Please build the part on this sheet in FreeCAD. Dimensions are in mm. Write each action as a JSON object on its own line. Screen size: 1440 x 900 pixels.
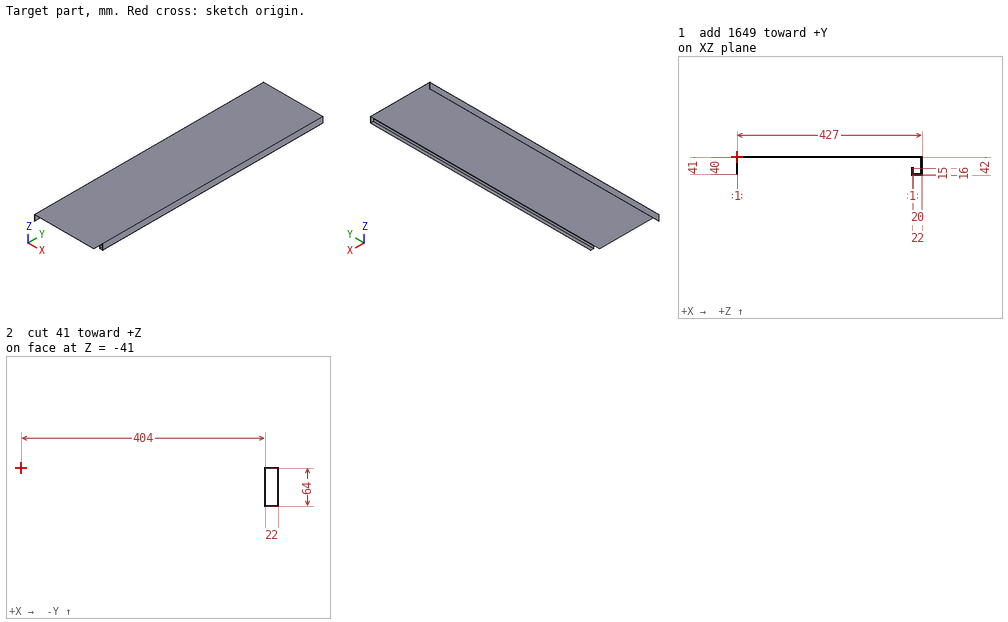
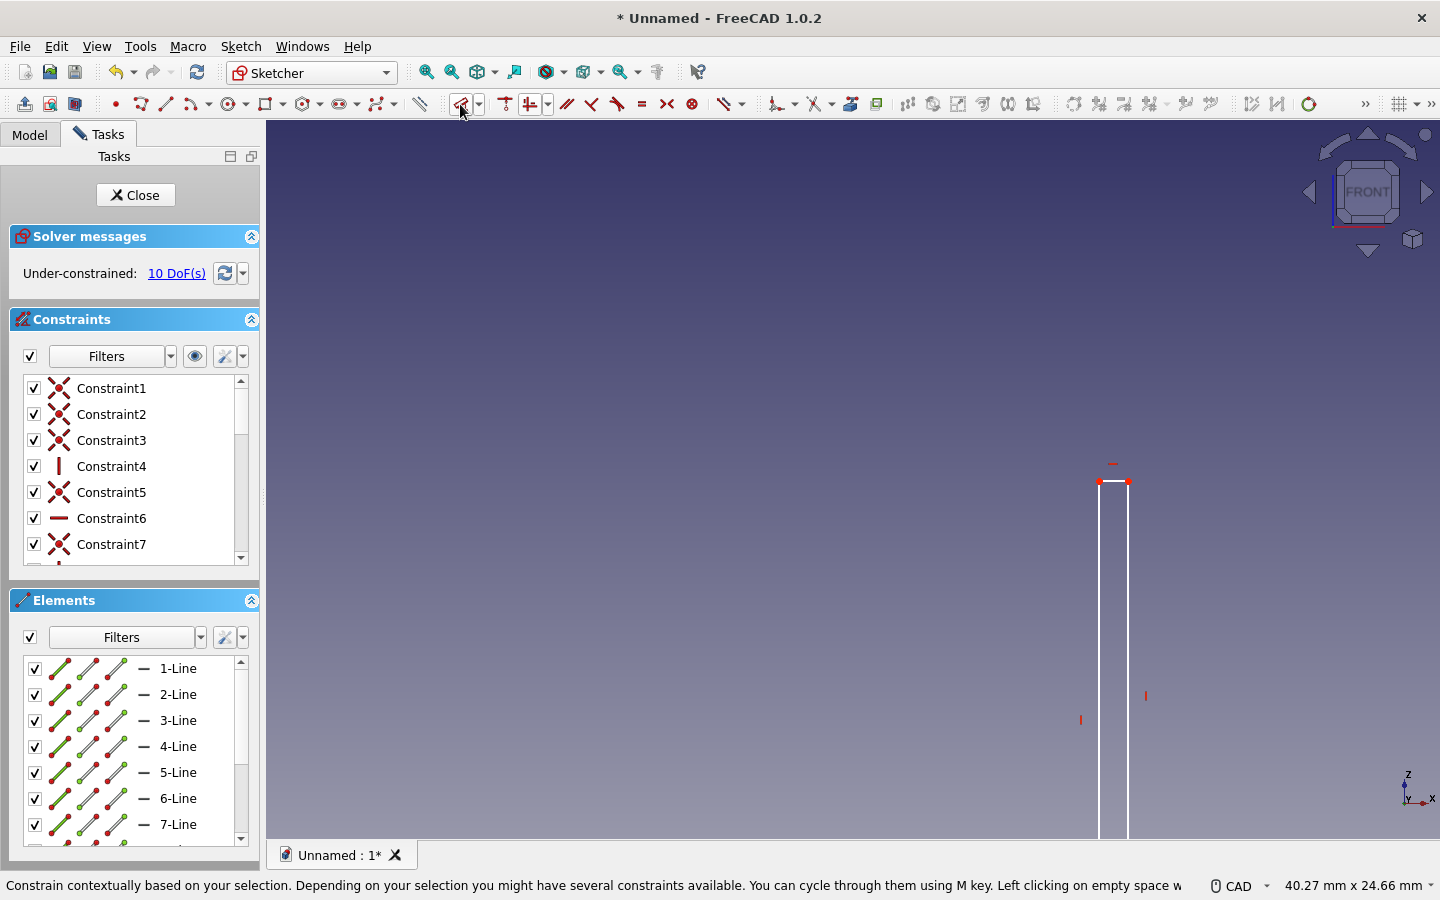
{"action": "scroll", "coordinate": [1126, 490], "scroll_direction": "down", "scroll_amount": 14}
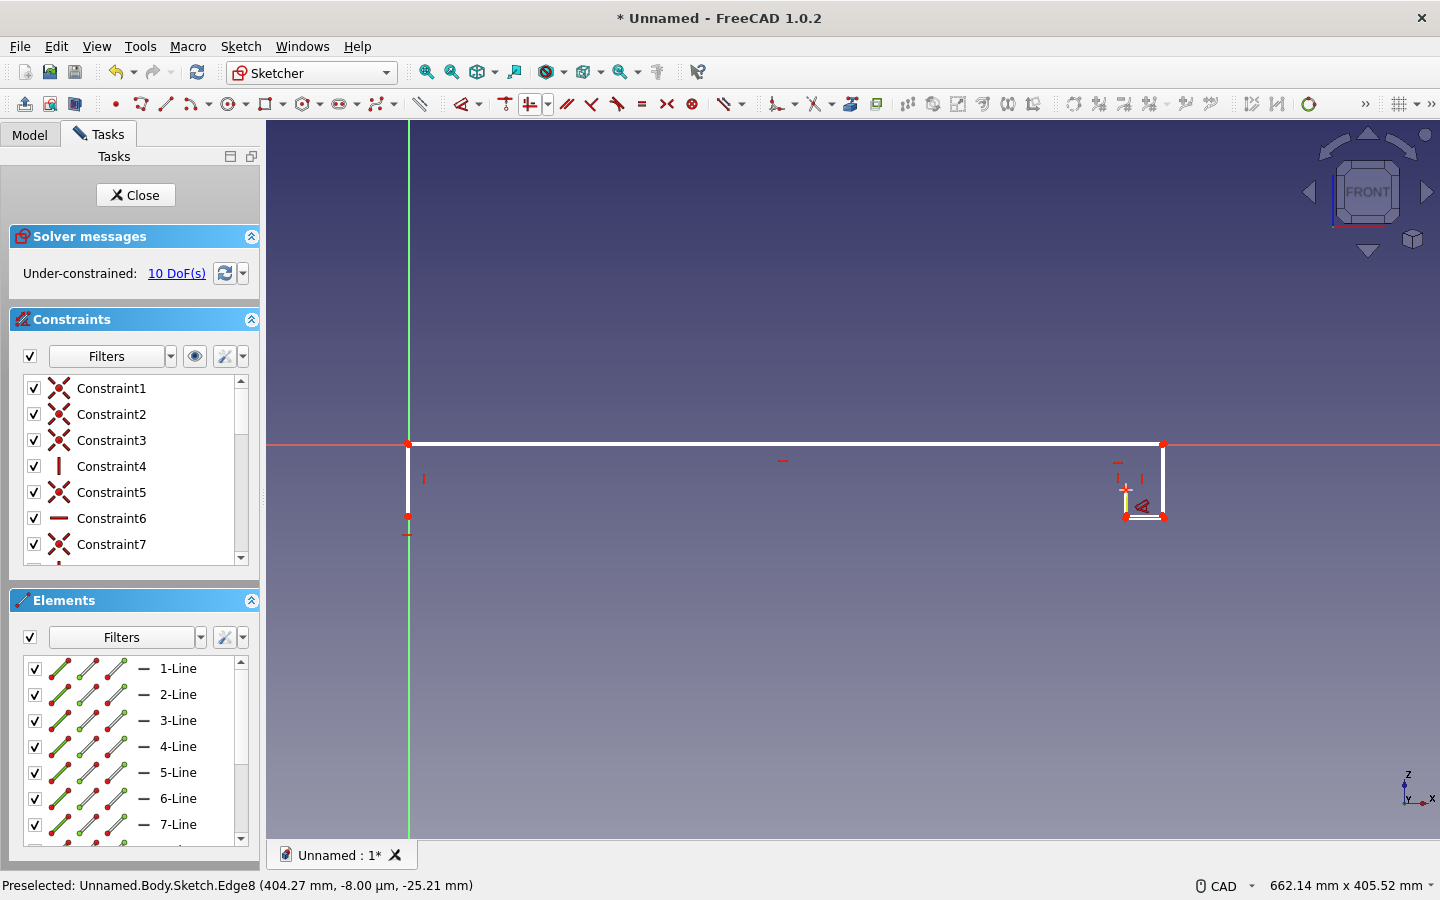
{"action": "scroll", "coordinate": [408, 517], "scroll_direction": "up", "scroll_amount": 16}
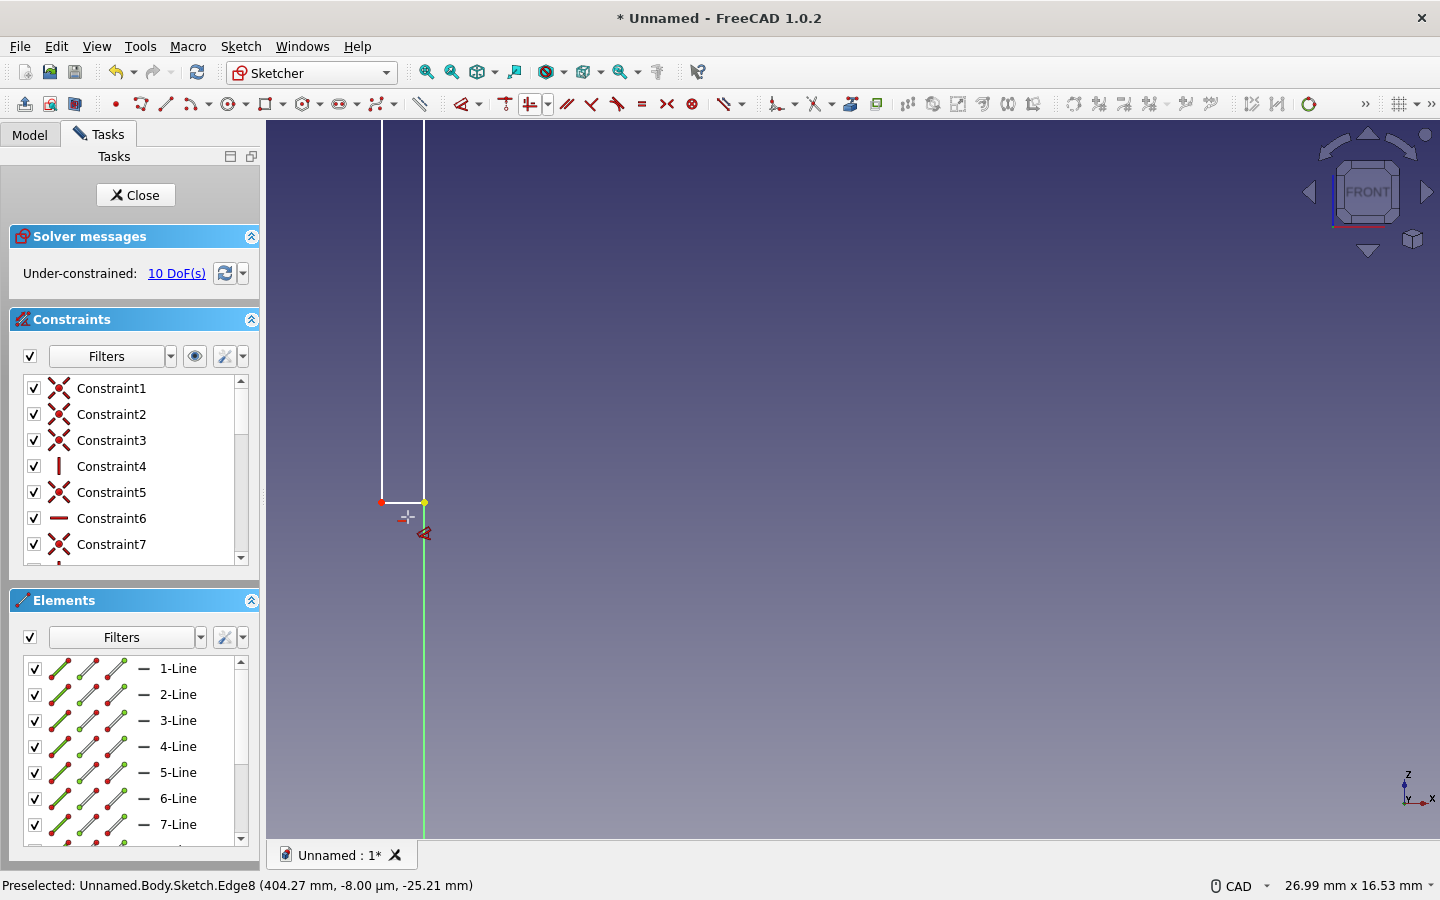
{"action": "left_click", "coordinate": [407, 503]}
{"action": "left_click", "coordinate": [403, 537]}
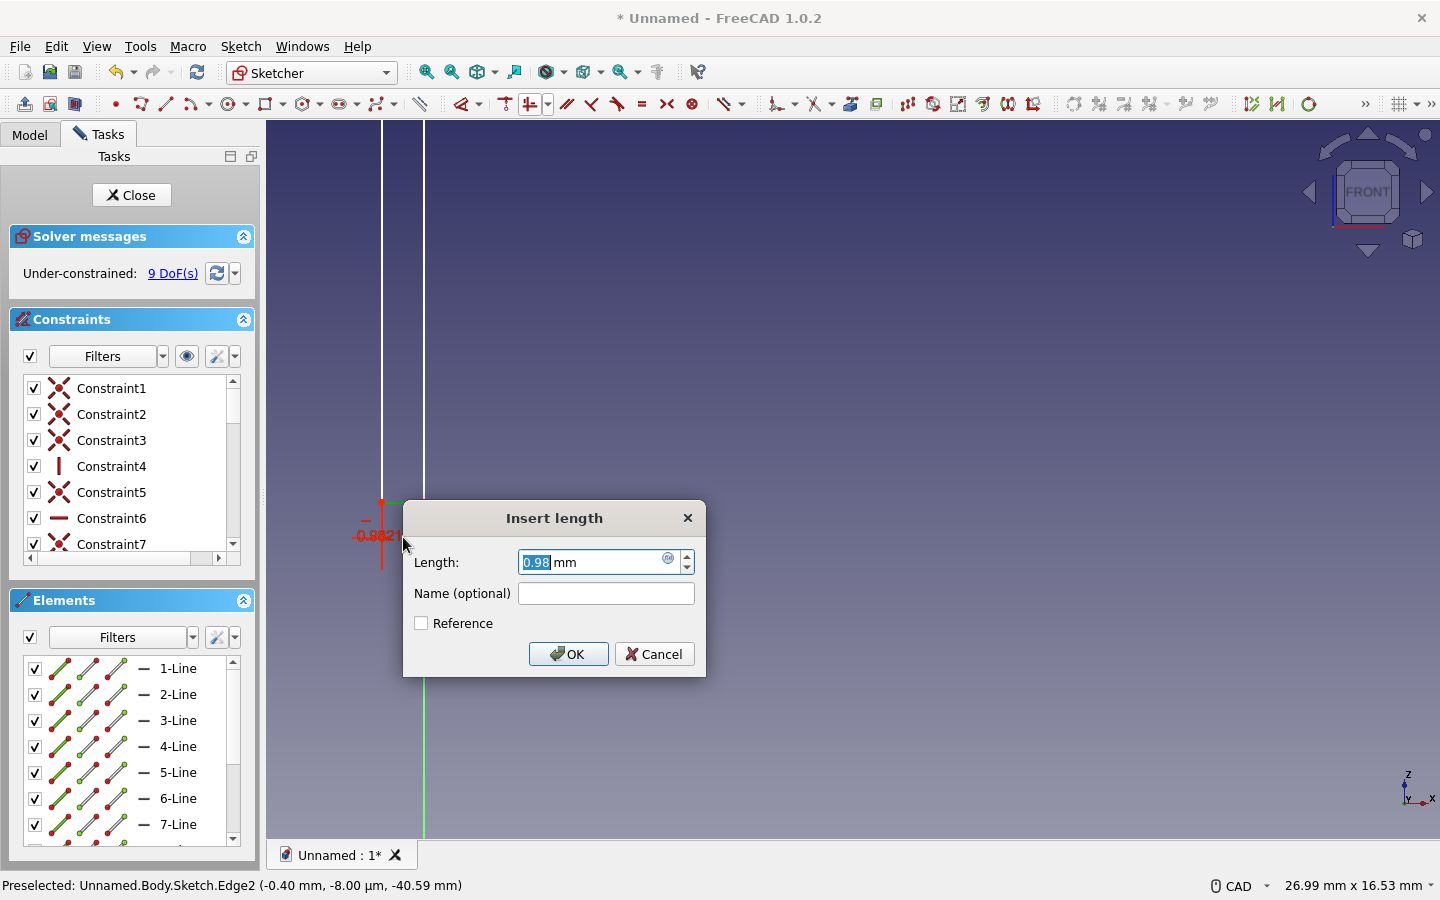
{"action": "type", "text": "1"}
{"action": "key", "text": "Return"}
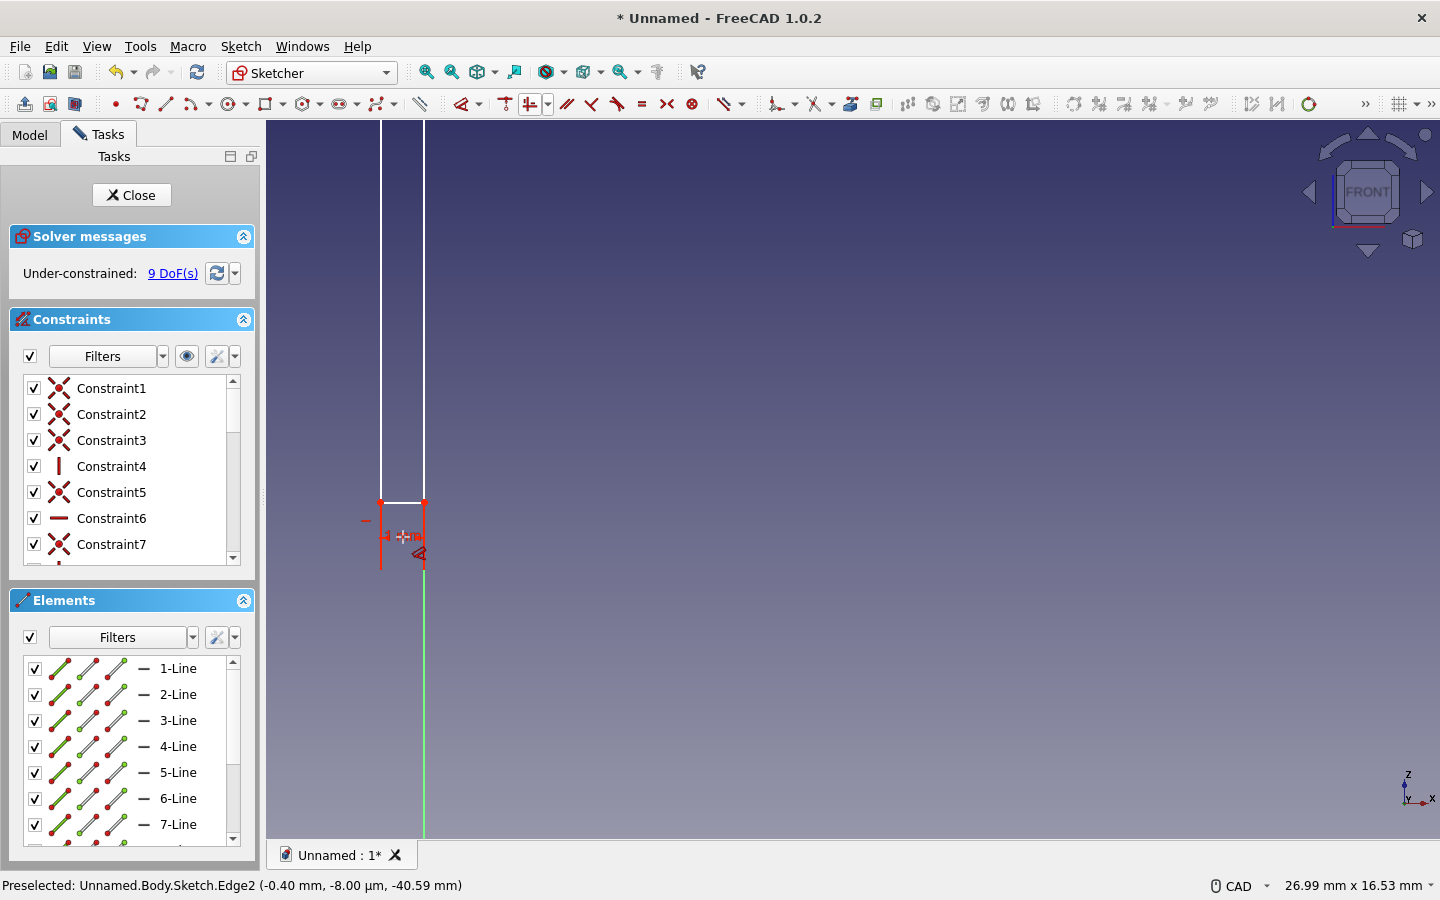
{"action": "scroll", "coordinate": [319, 525], "scroll_direction": "down", "scroll_amount": 15}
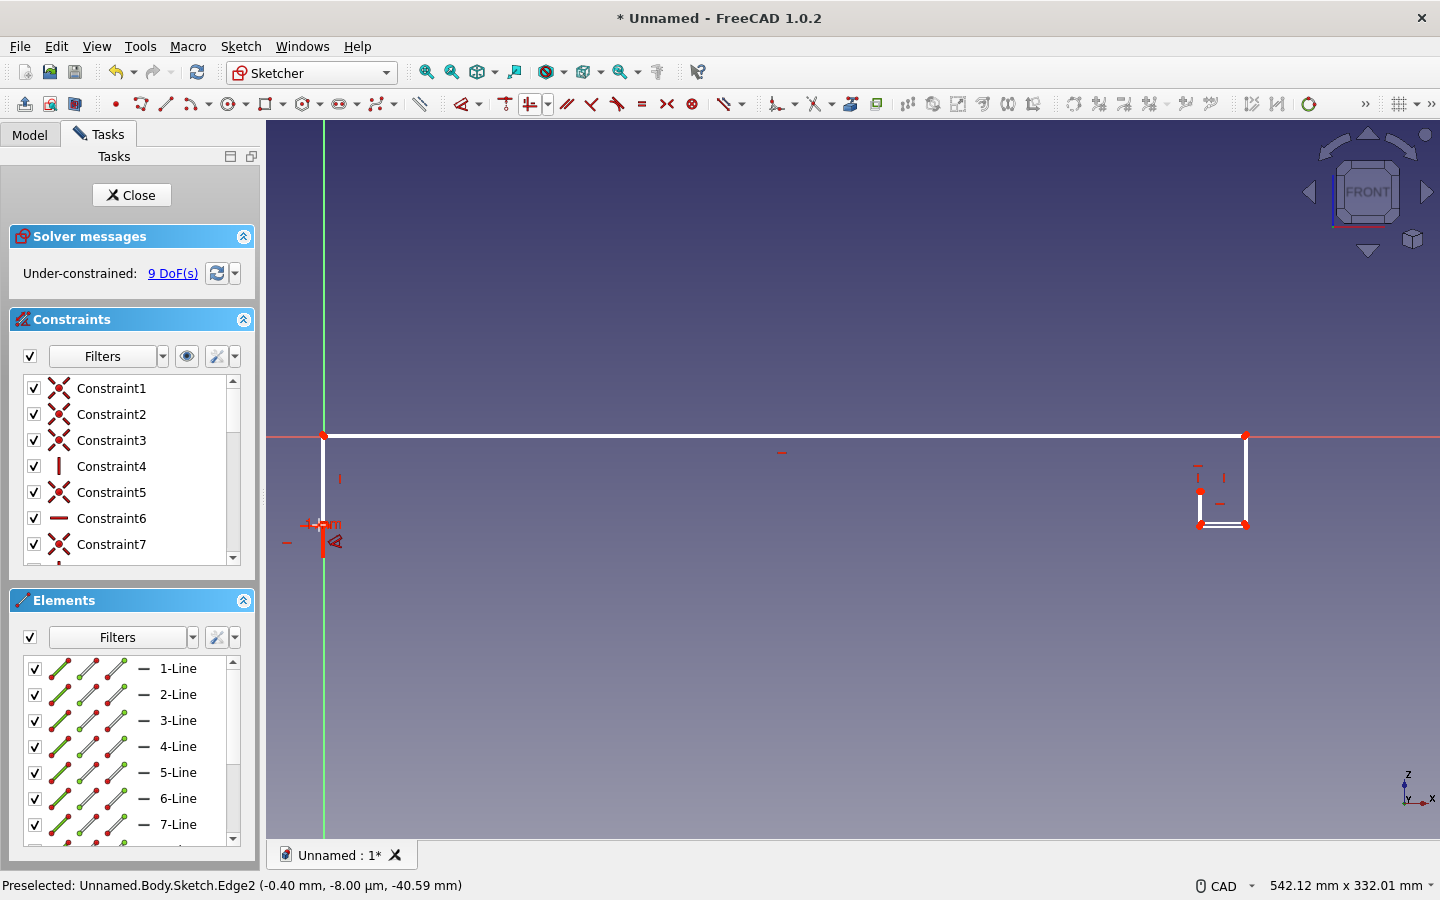
{"action": "scroll", "coordinate": [1200, 491], "scroll_direction": "up", "scroll_amount": 15}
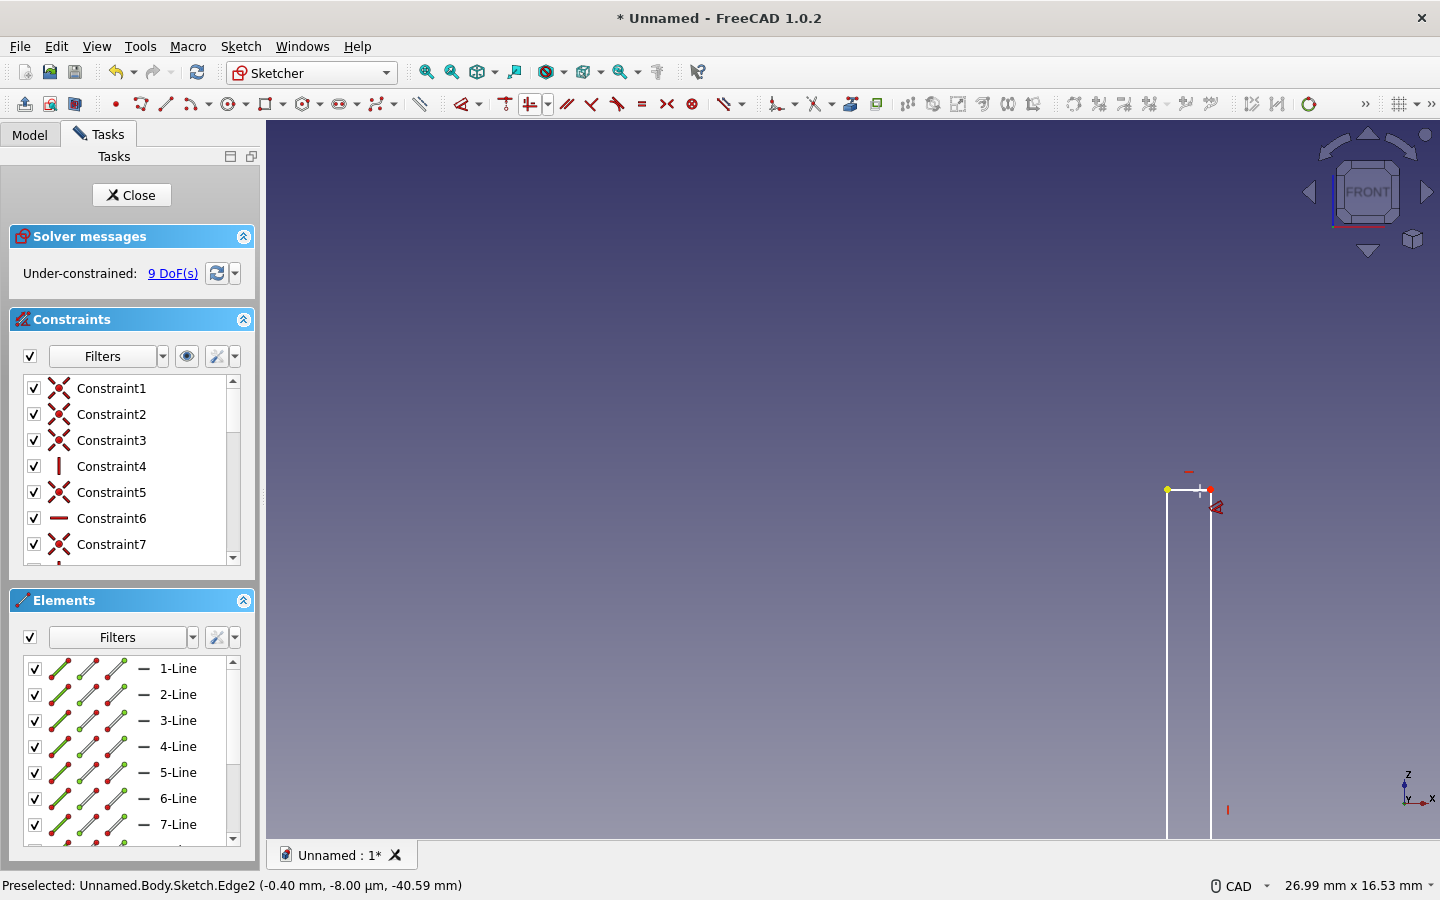
{"action": "left_click", "coordinate": [1180, 490]}
{"action": "left_click", "coordinate": [1189, 524]}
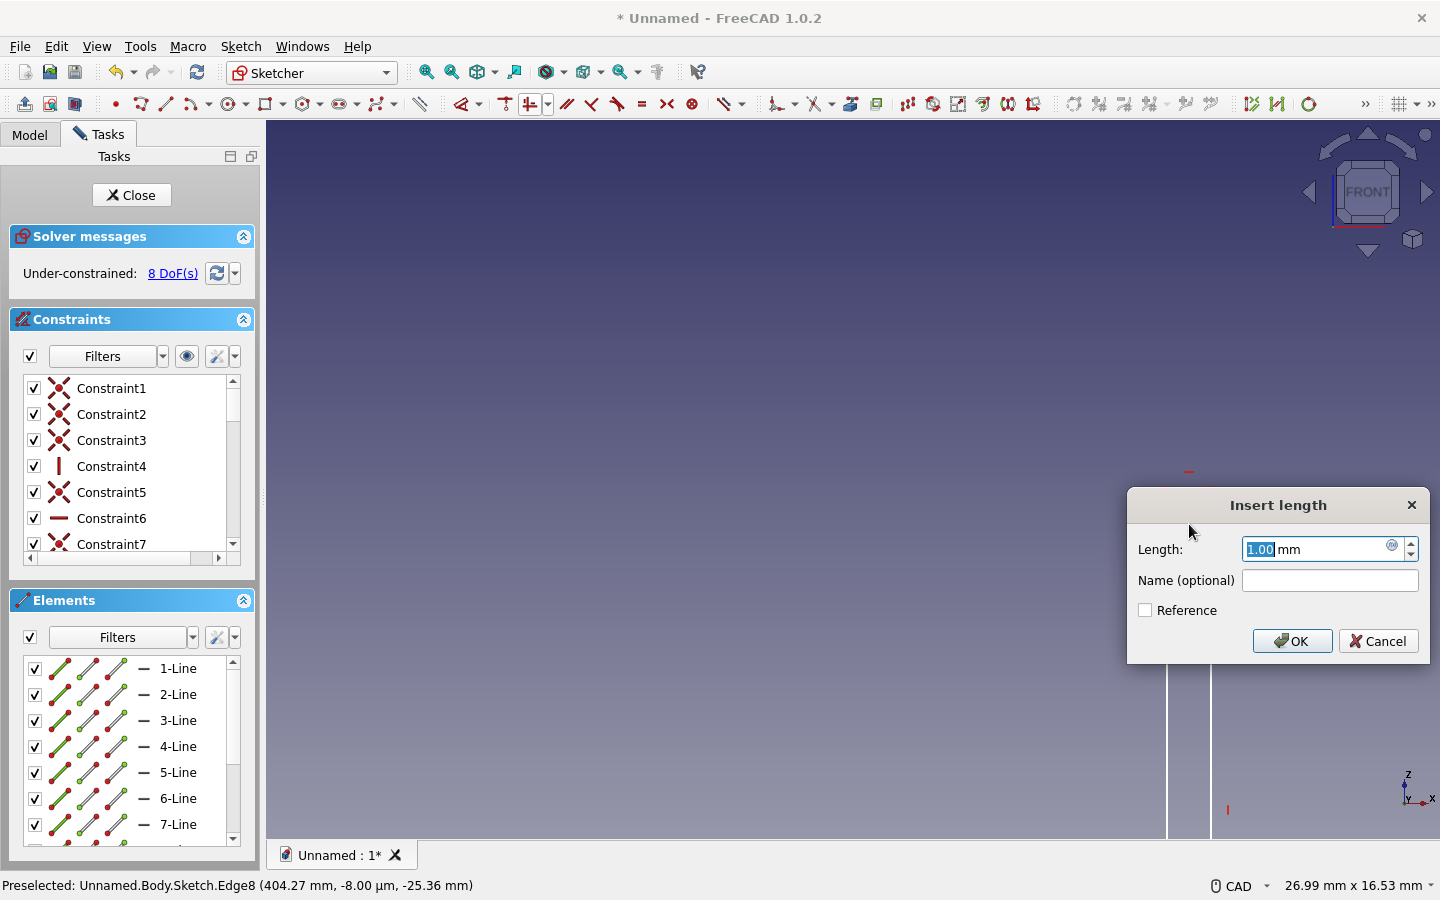
{"action": "type", "text": "1"}
{"action": "key", "text": "Return"}